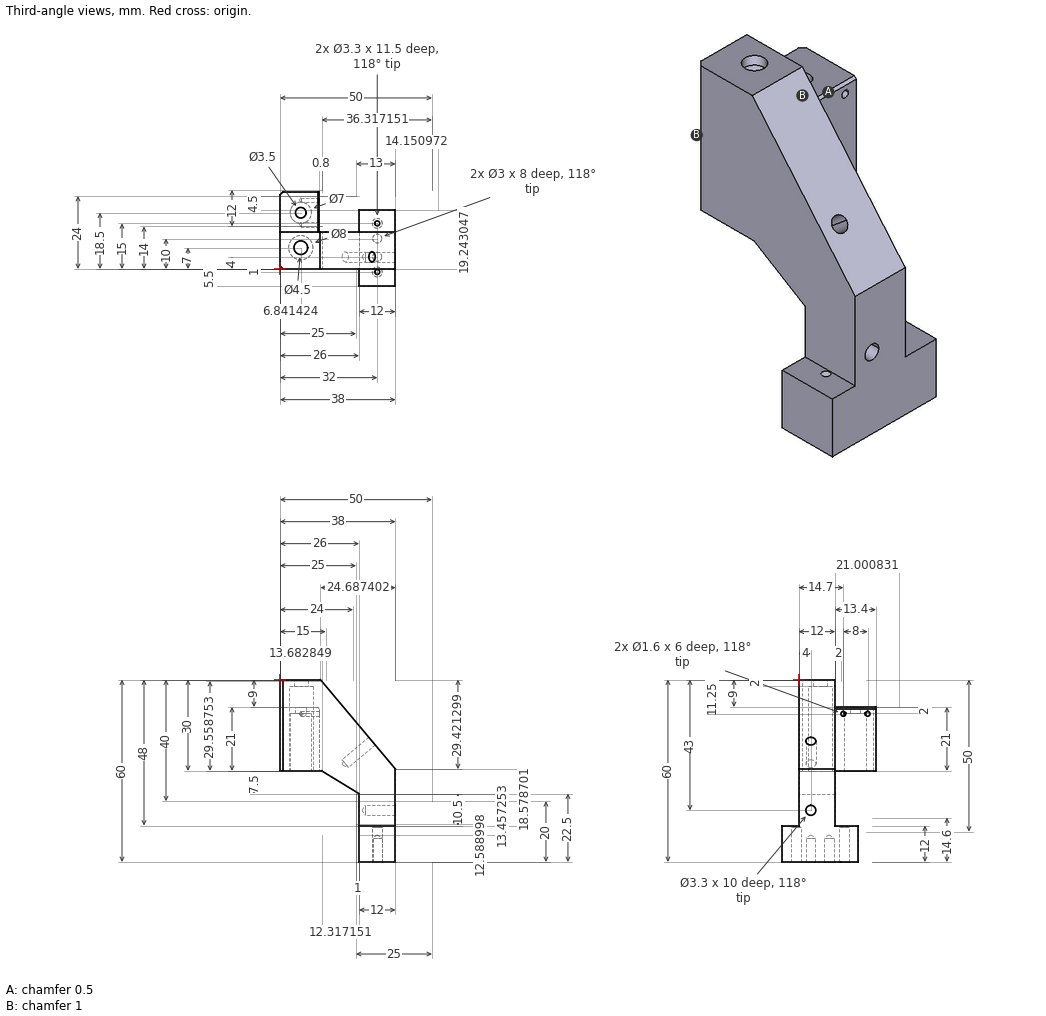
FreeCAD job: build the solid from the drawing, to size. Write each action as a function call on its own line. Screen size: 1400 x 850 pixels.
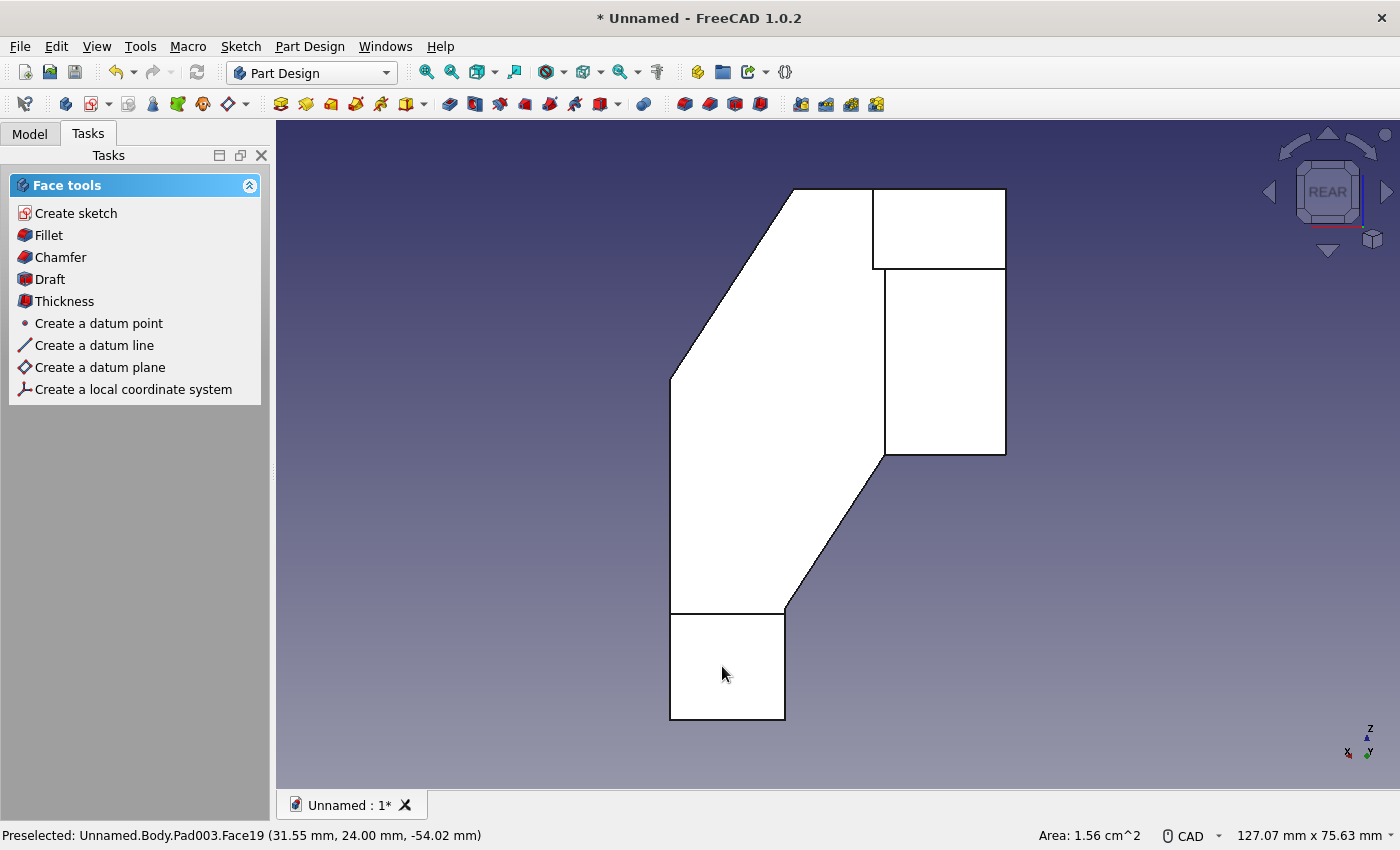
click(90, 104)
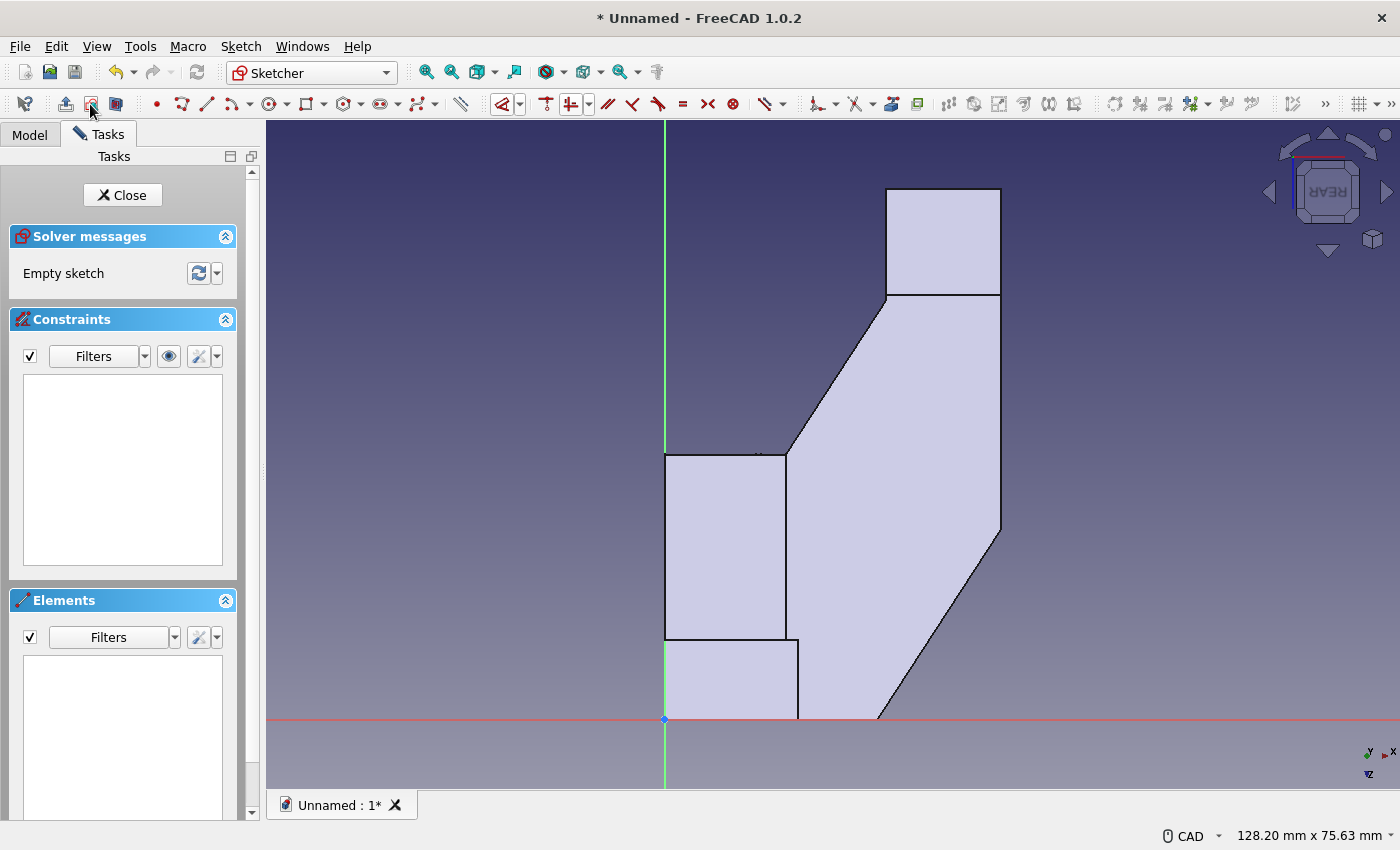
key(q)
key(s)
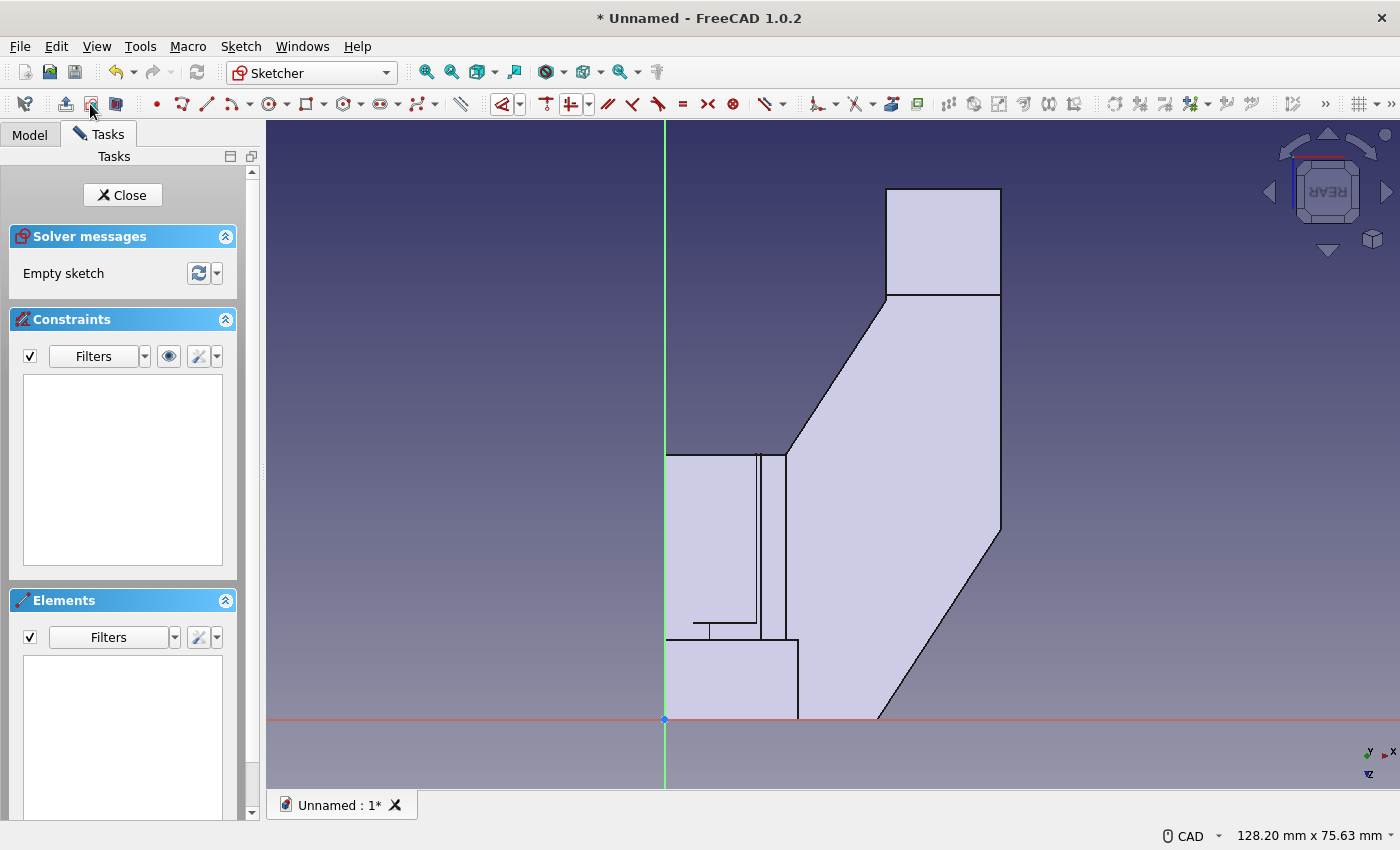
scroll(993, 153, up, 4)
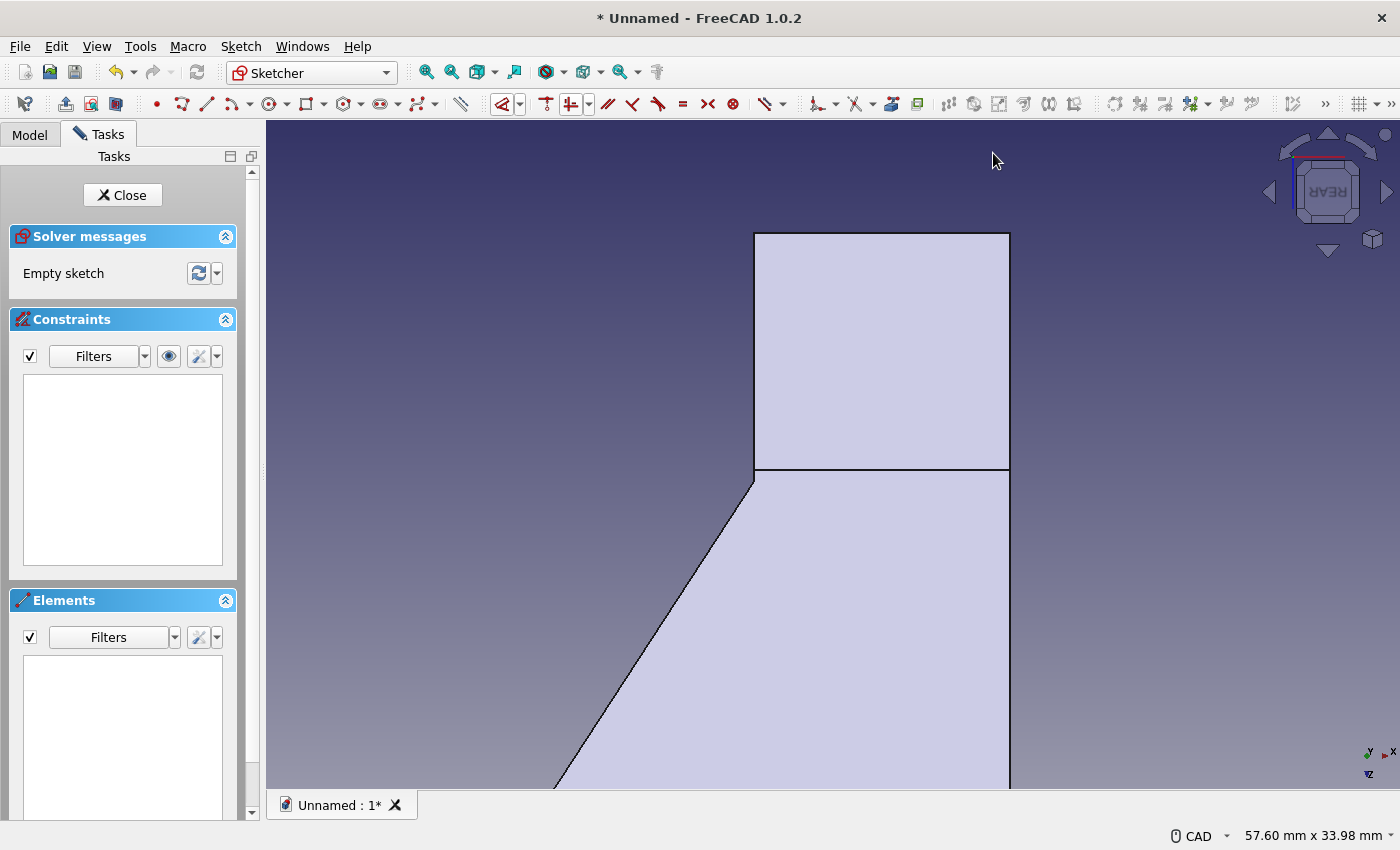
click(306, 104)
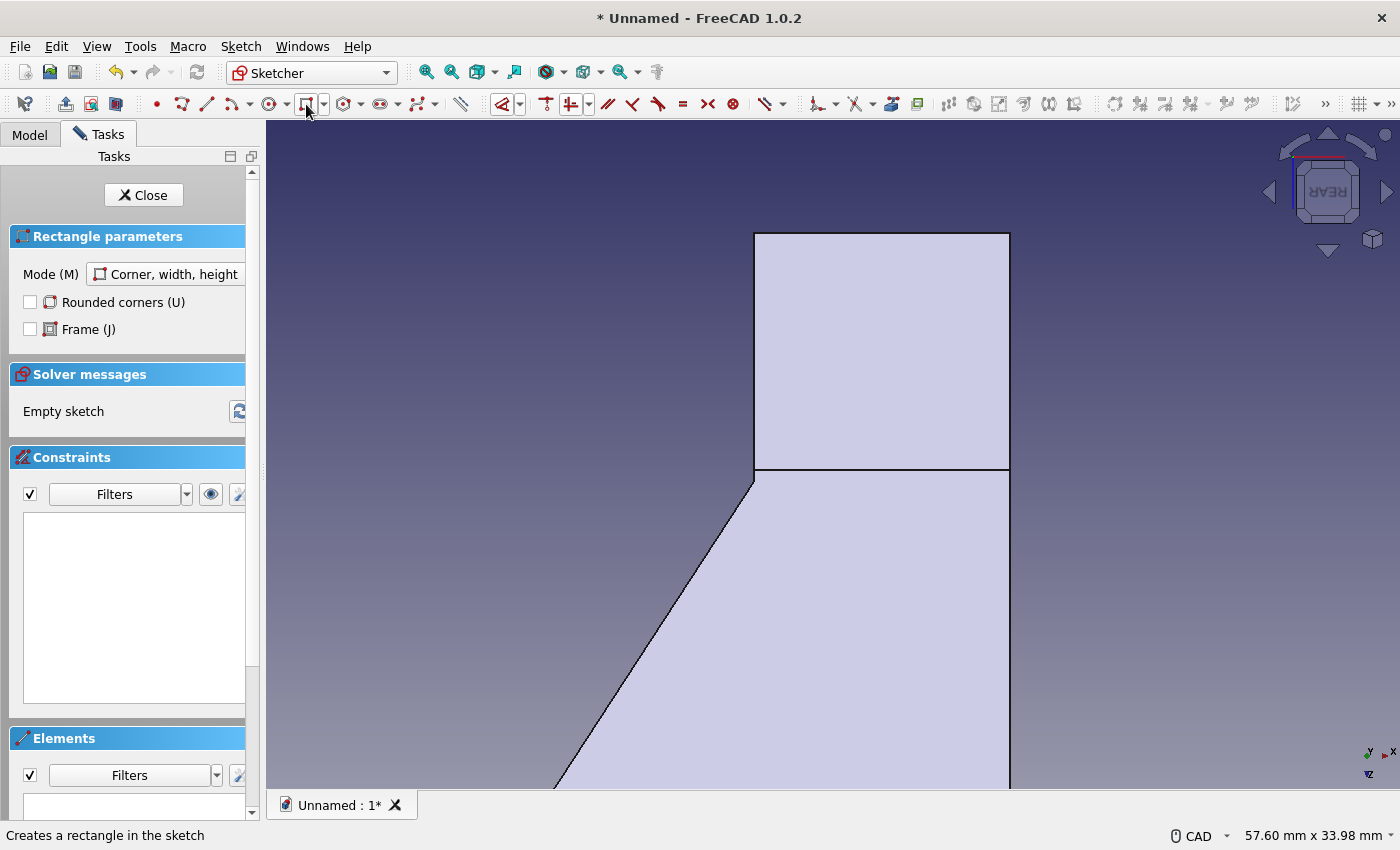
click(754, 233)
click(774, 676)
key(Escape)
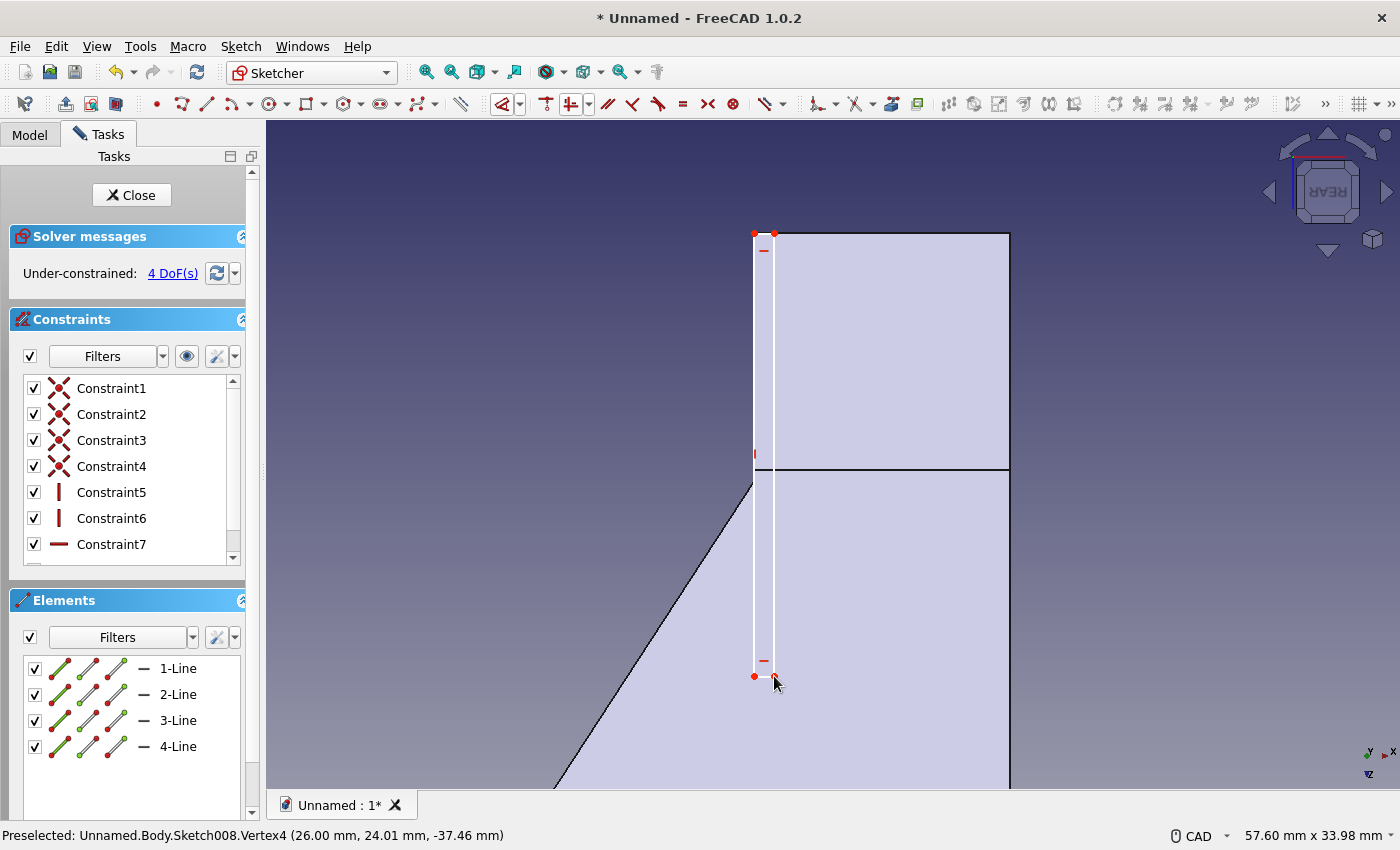
scroll(764, 677, up, 4)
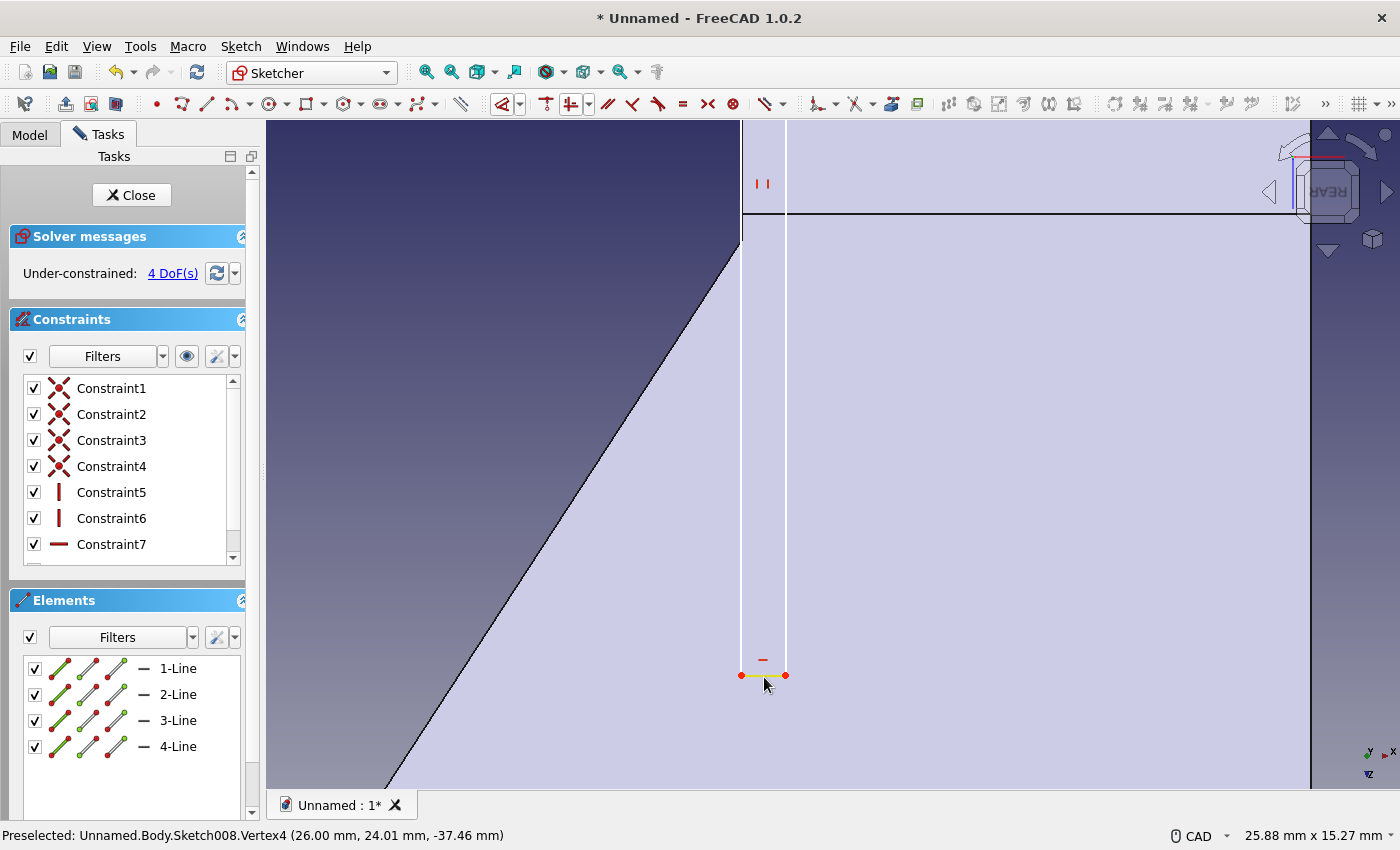
click(763, 676)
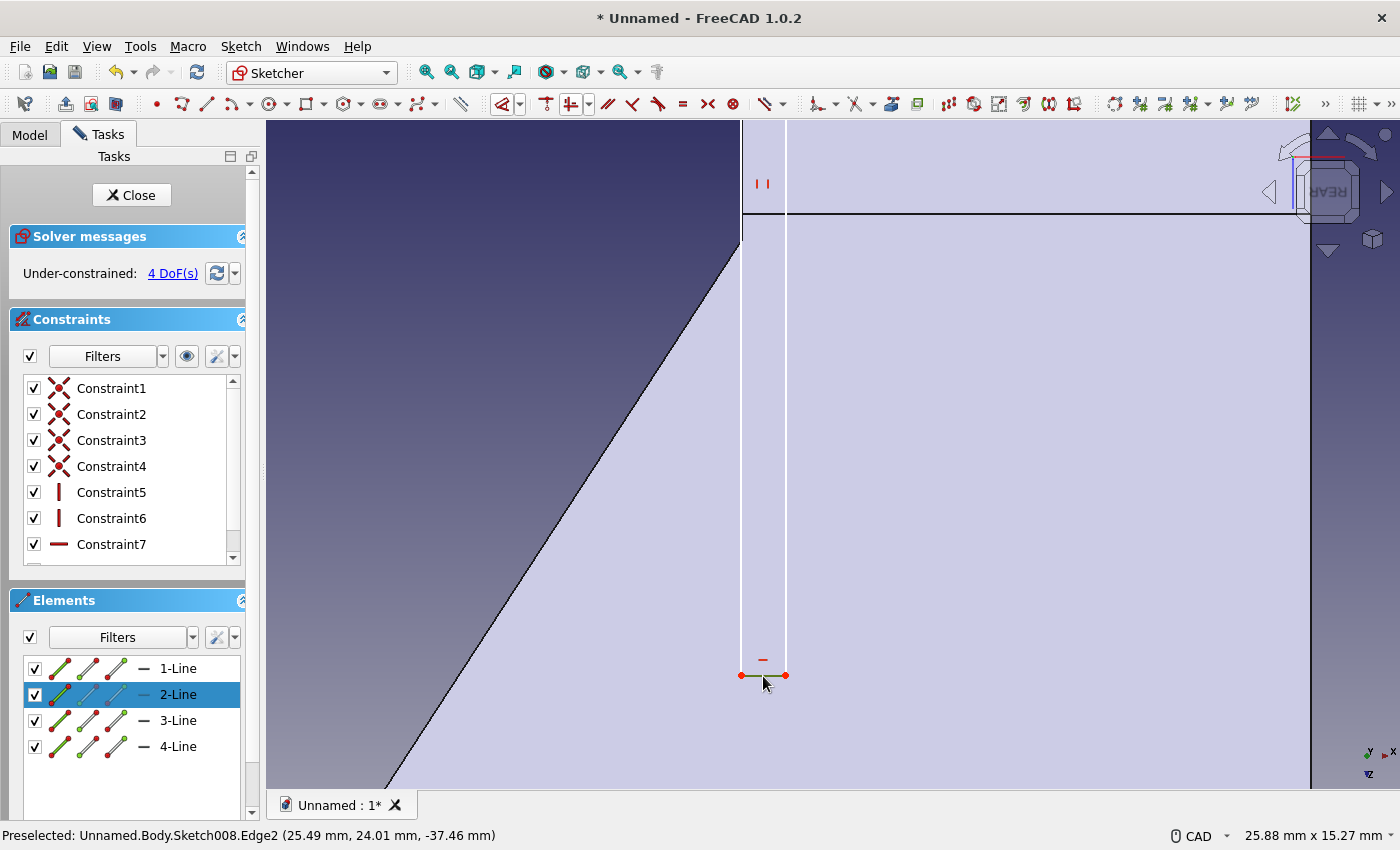
click(520, 104)